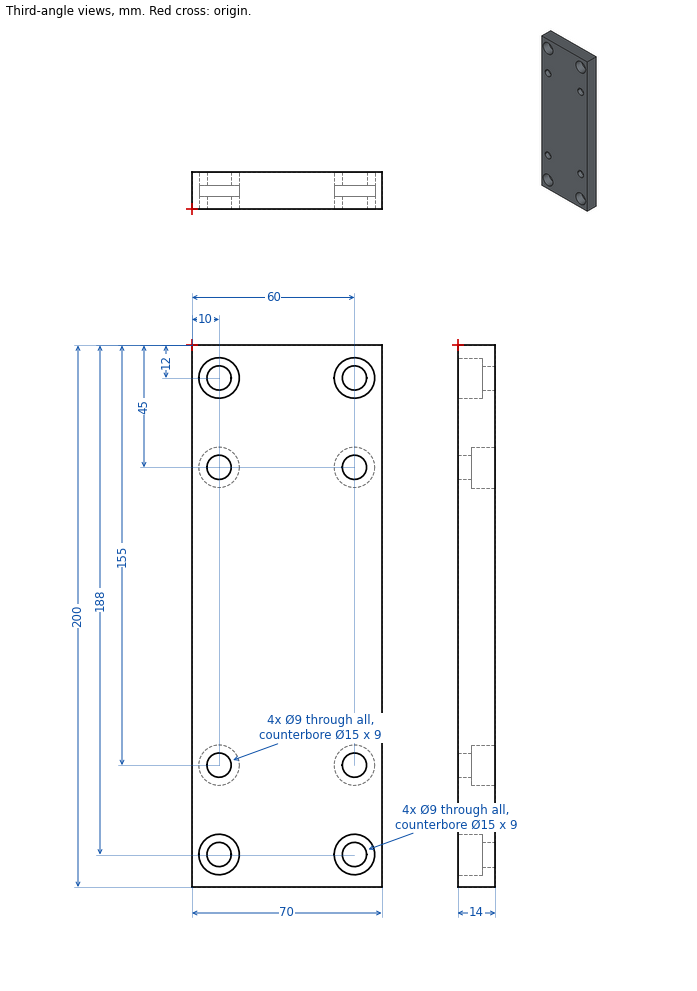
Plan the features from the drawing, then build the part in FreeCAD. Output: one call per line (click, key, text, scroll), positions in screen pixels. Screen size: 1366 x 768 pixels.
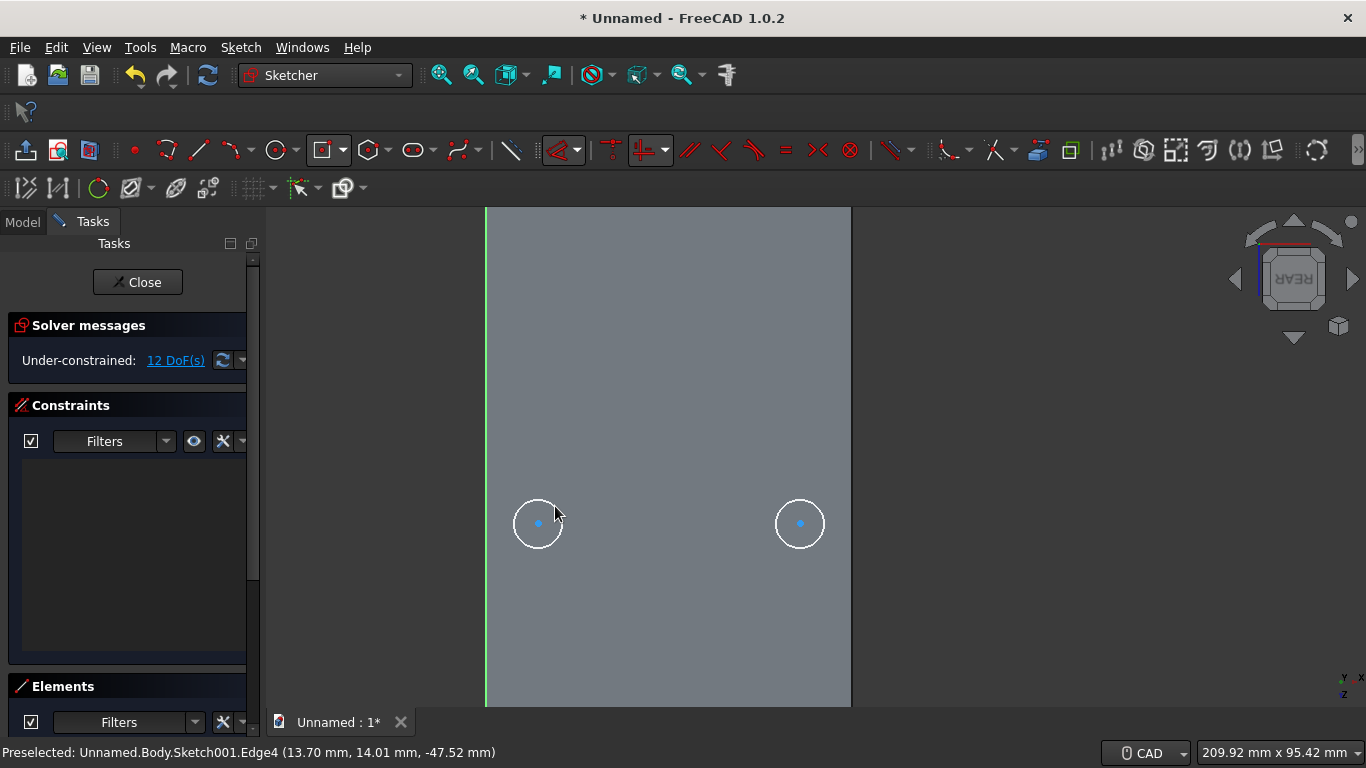
scroll(802, 525, down, 5)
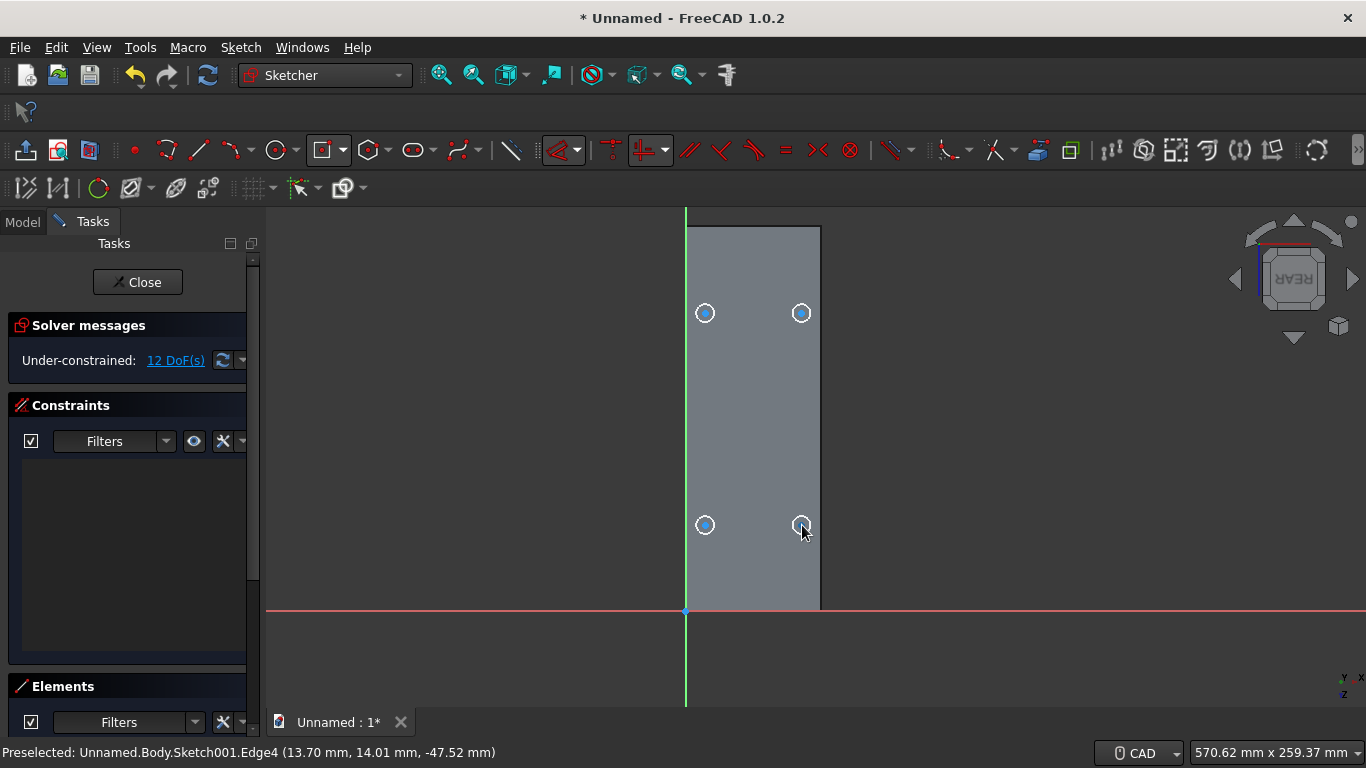
scroll(711, 307, up, 3)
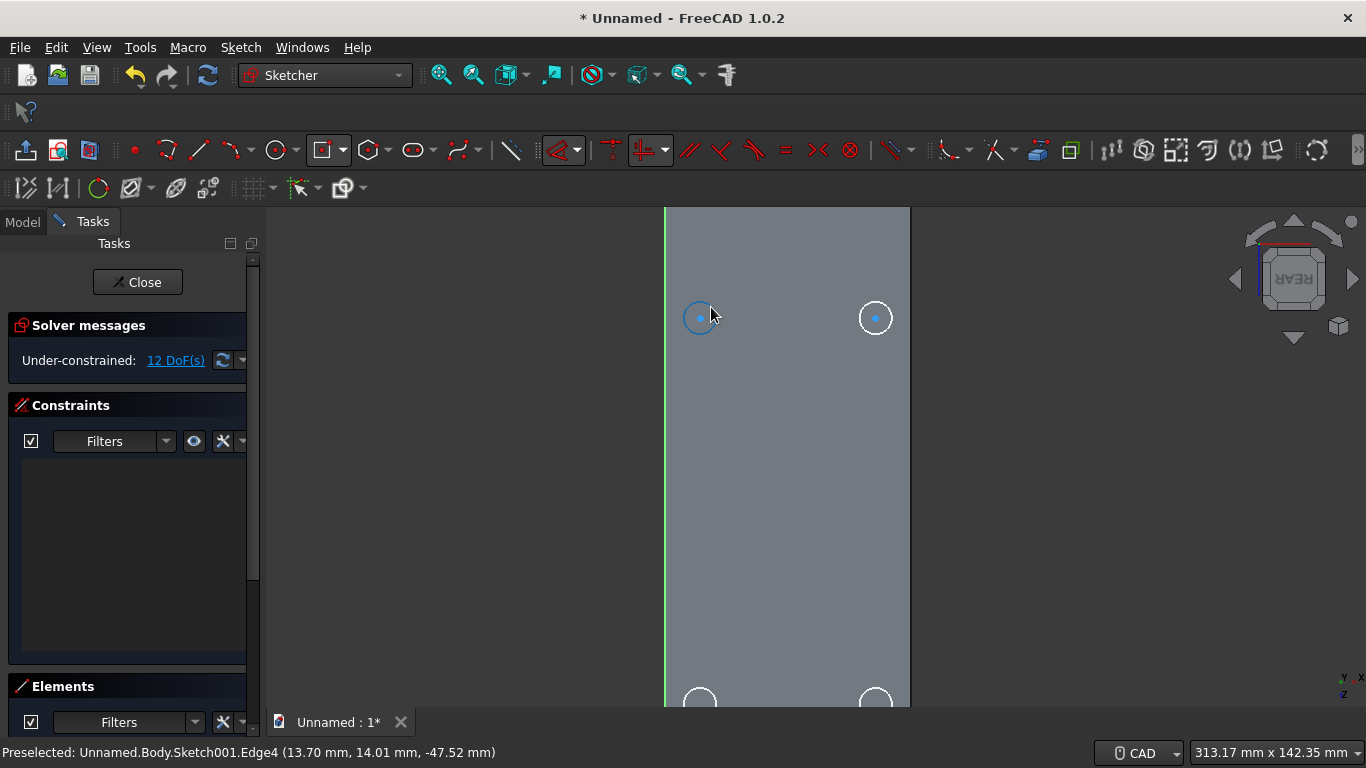
click(711, 307)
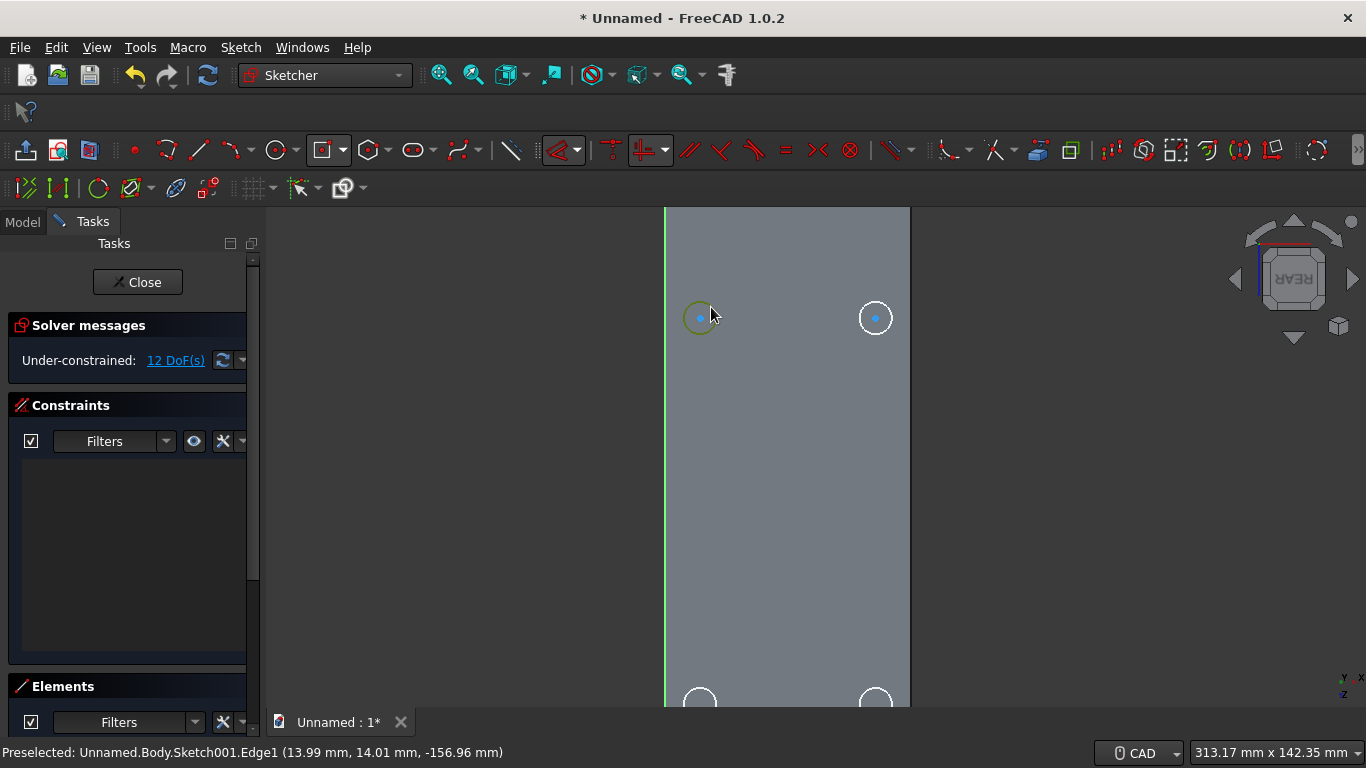
click(887, 307)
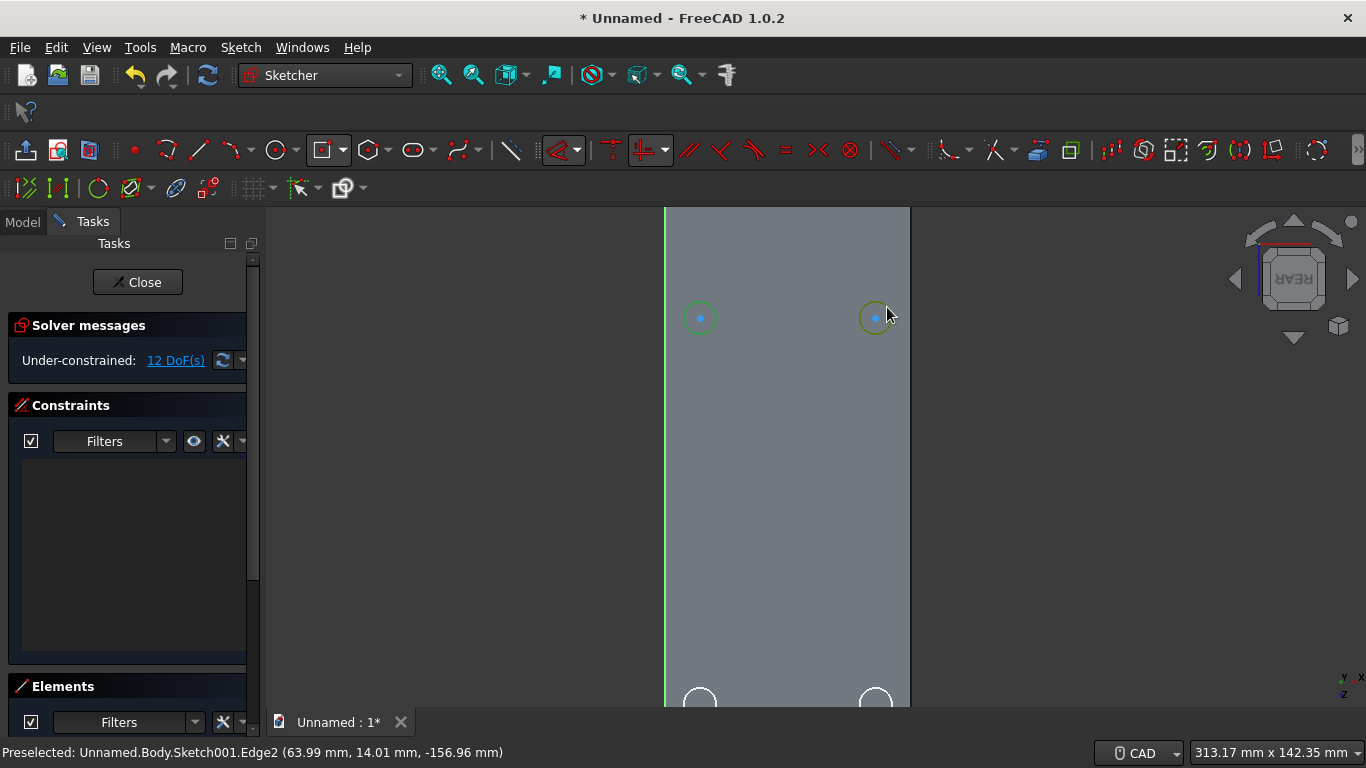
scroll(710, 306, down, 3)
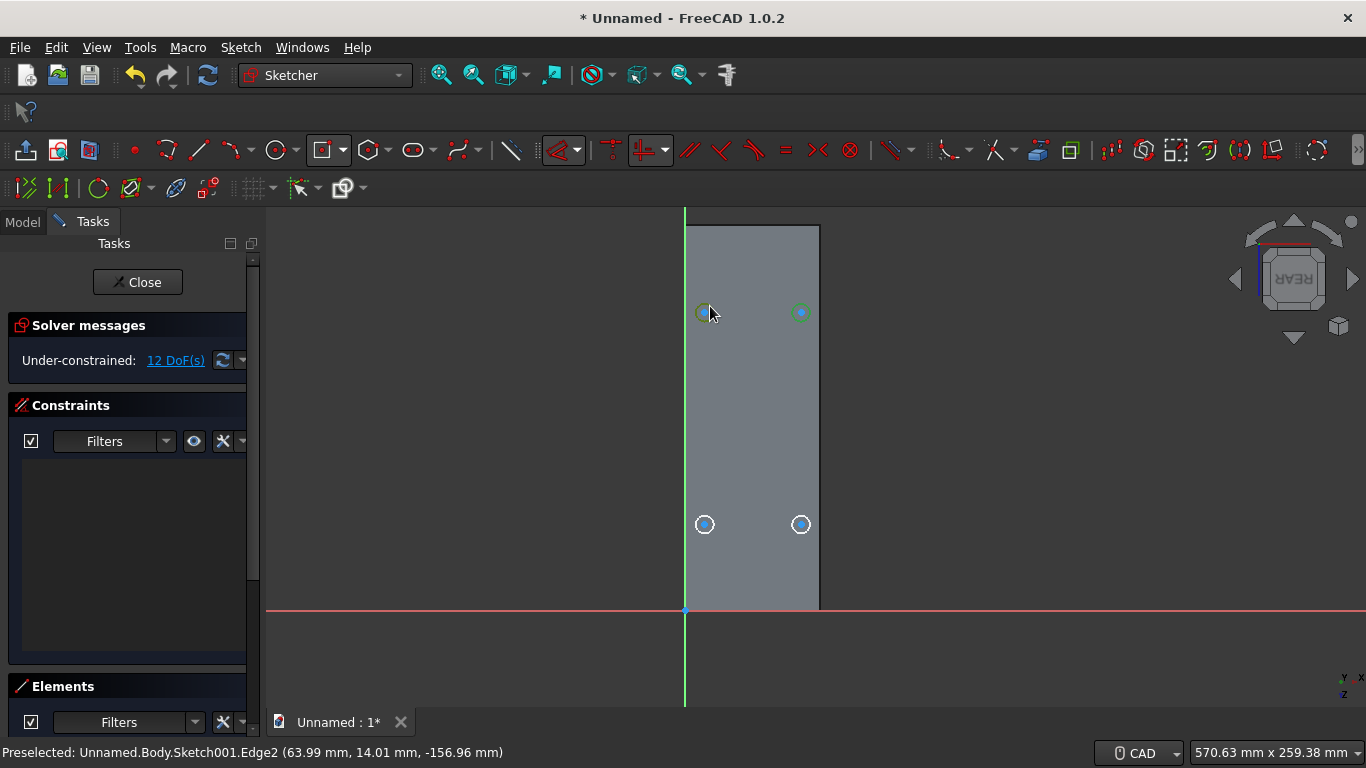
scroll(807, 518, up, 3)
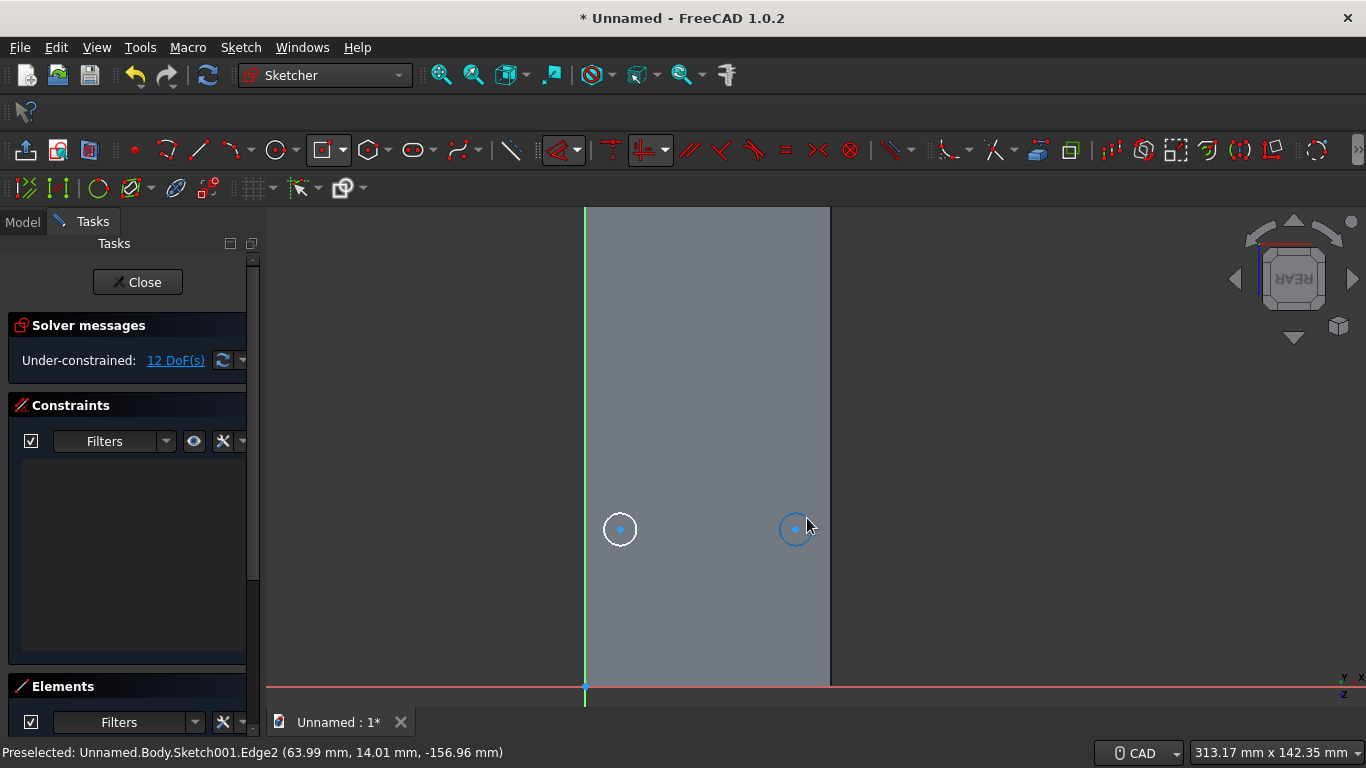
click(807, 518)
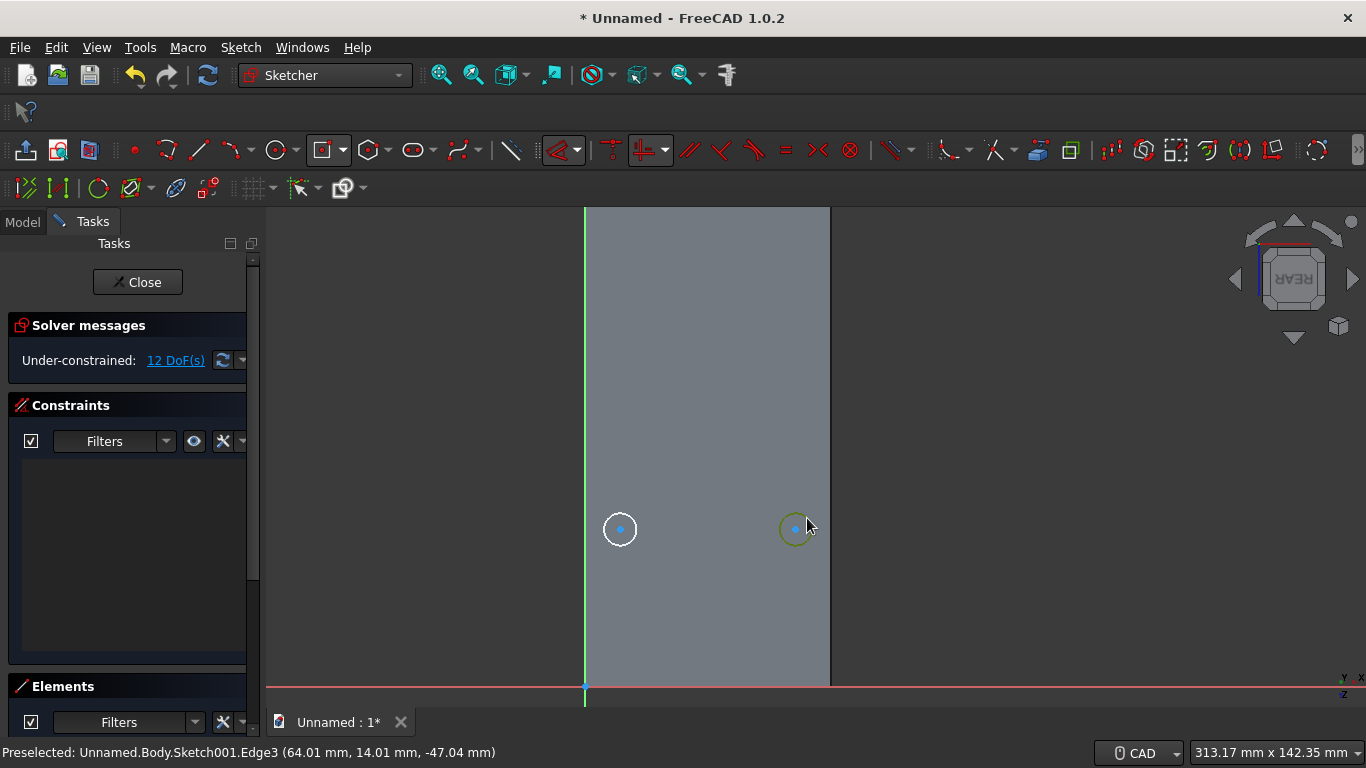
click(632, 518)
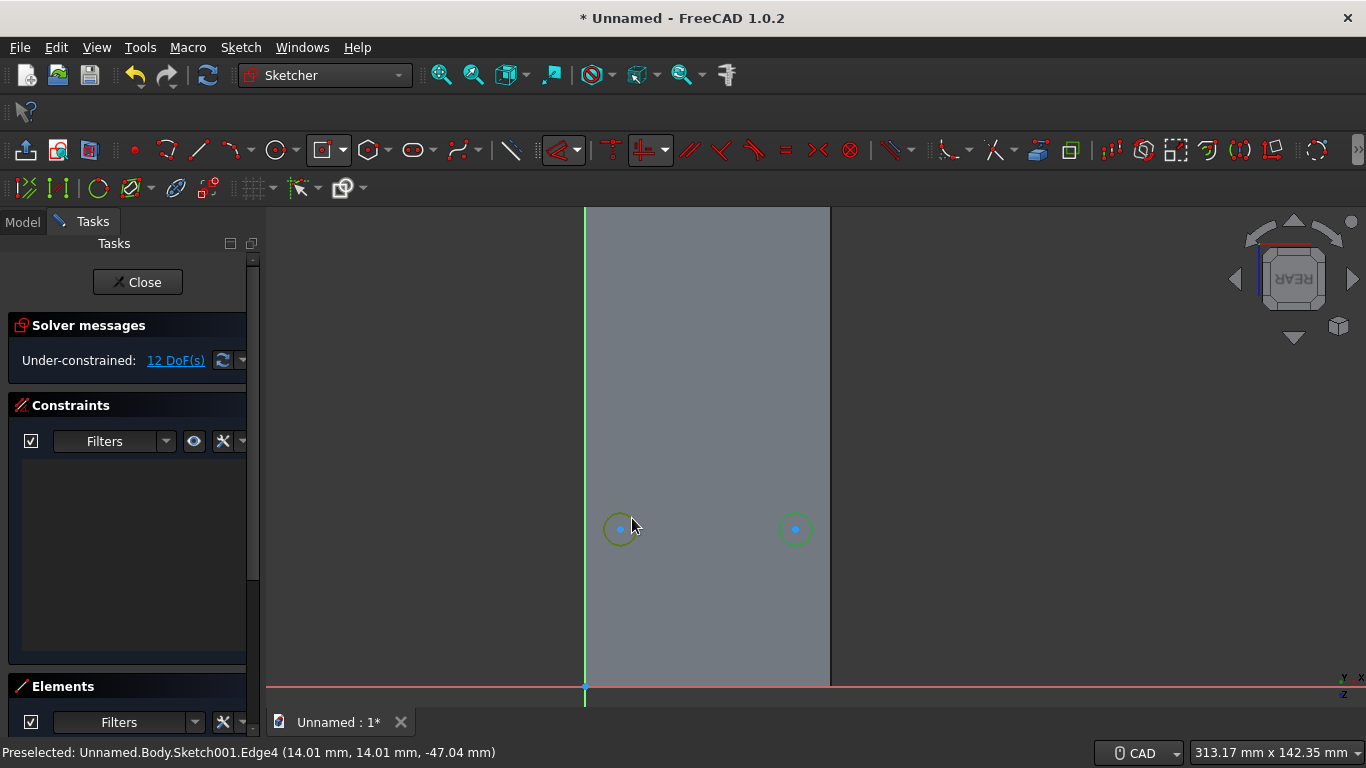
click(786, 150)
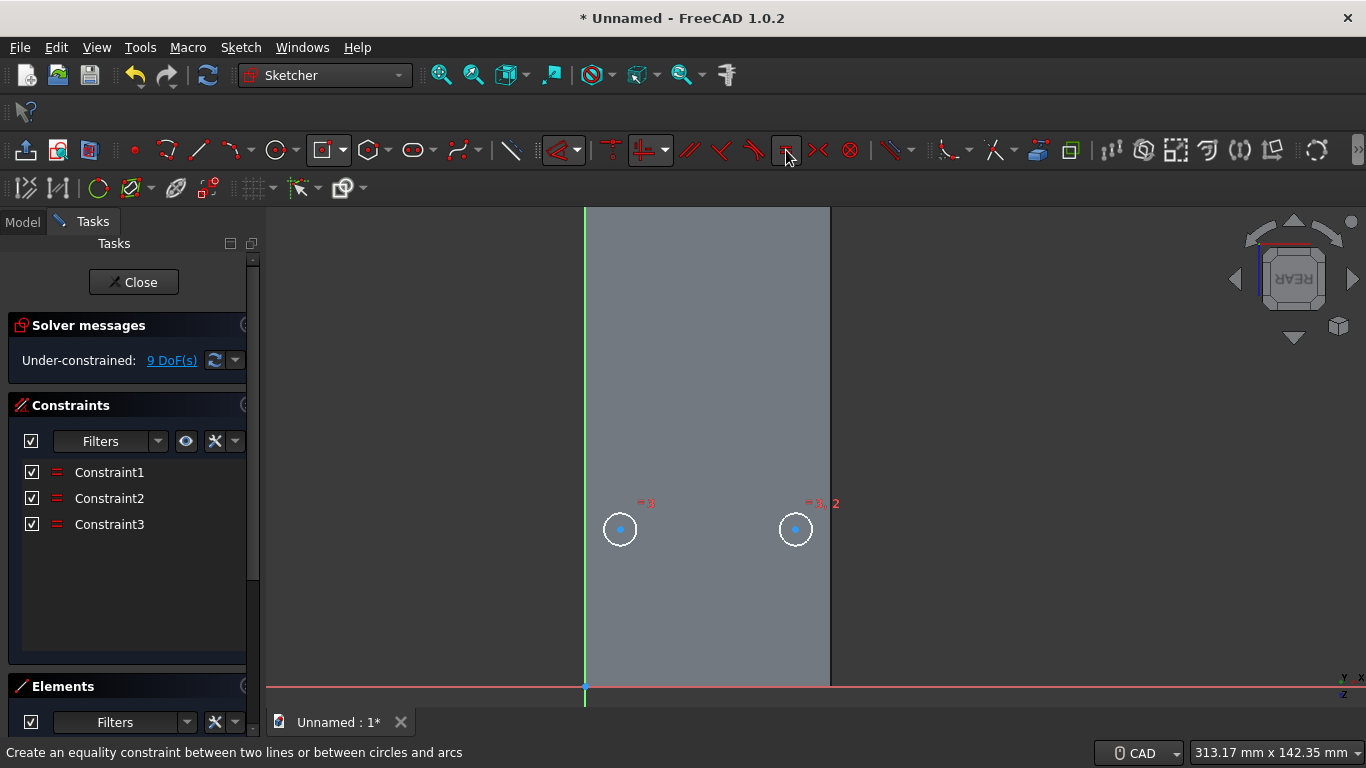
scroll(807, 518, down, 3)